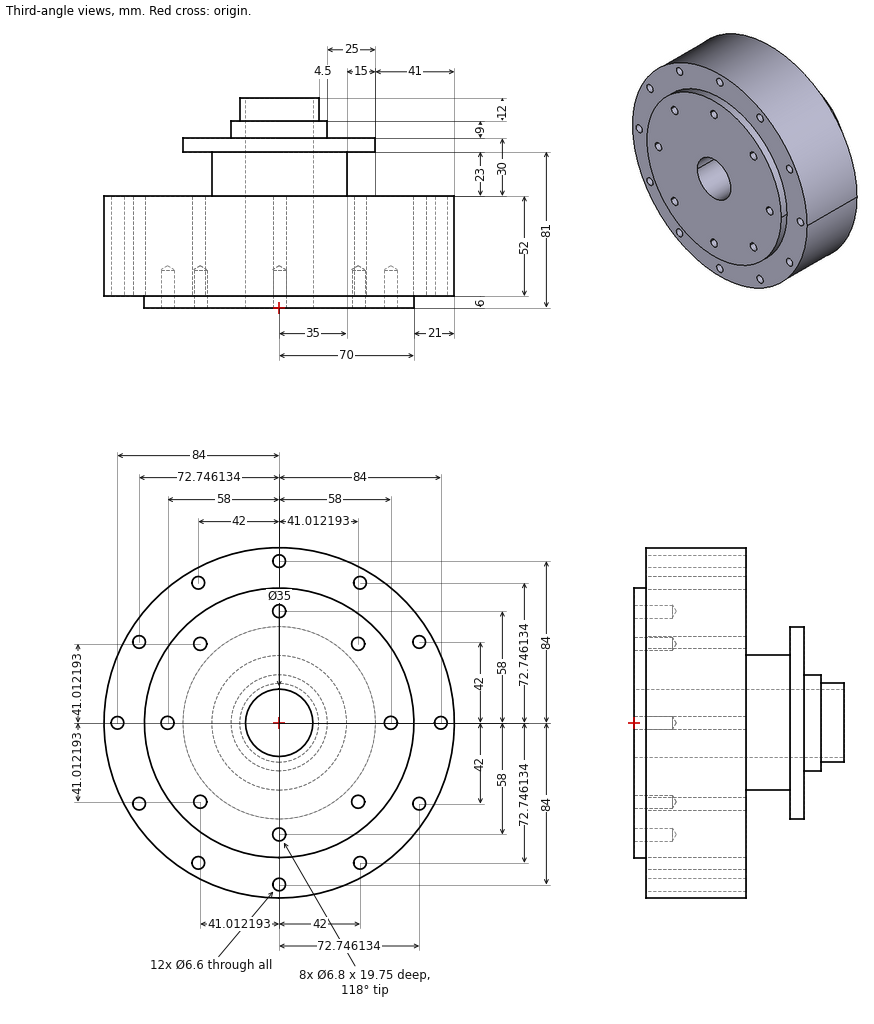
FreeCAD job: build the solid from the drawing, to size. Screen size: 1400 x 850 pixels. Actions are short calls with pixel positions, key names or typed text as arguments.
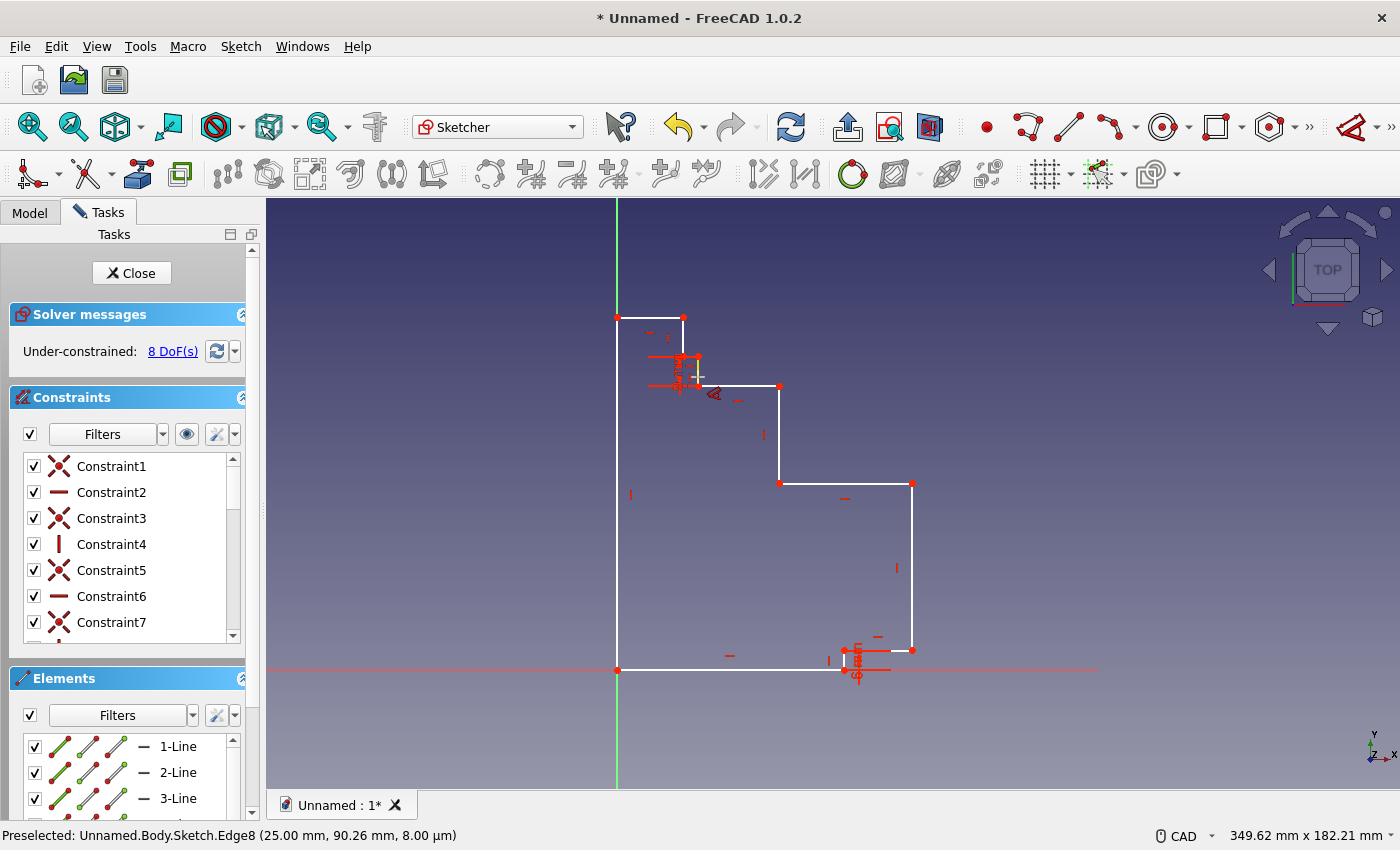
click(685, 670)
click(731, 704)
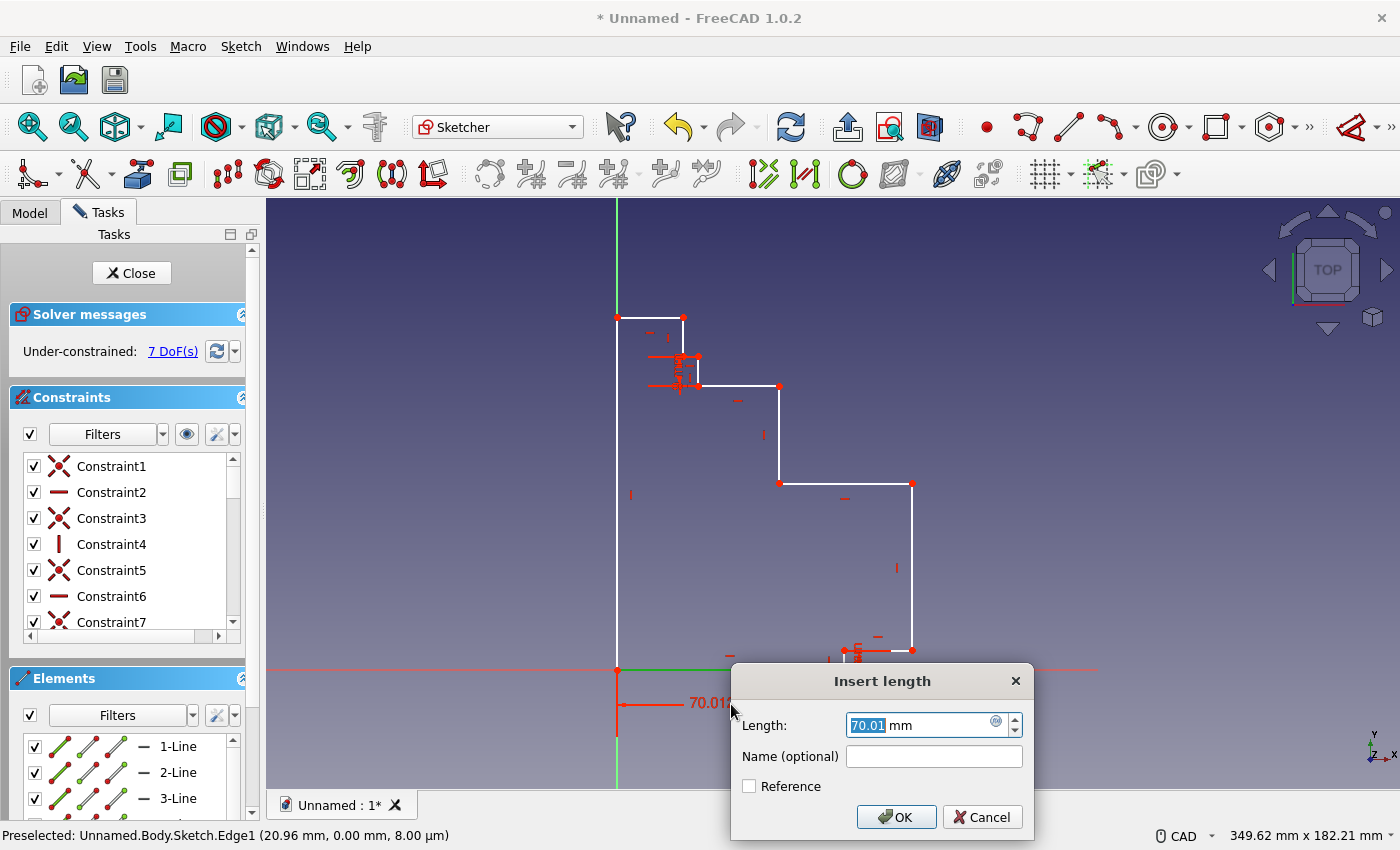
text(70)
key(Return)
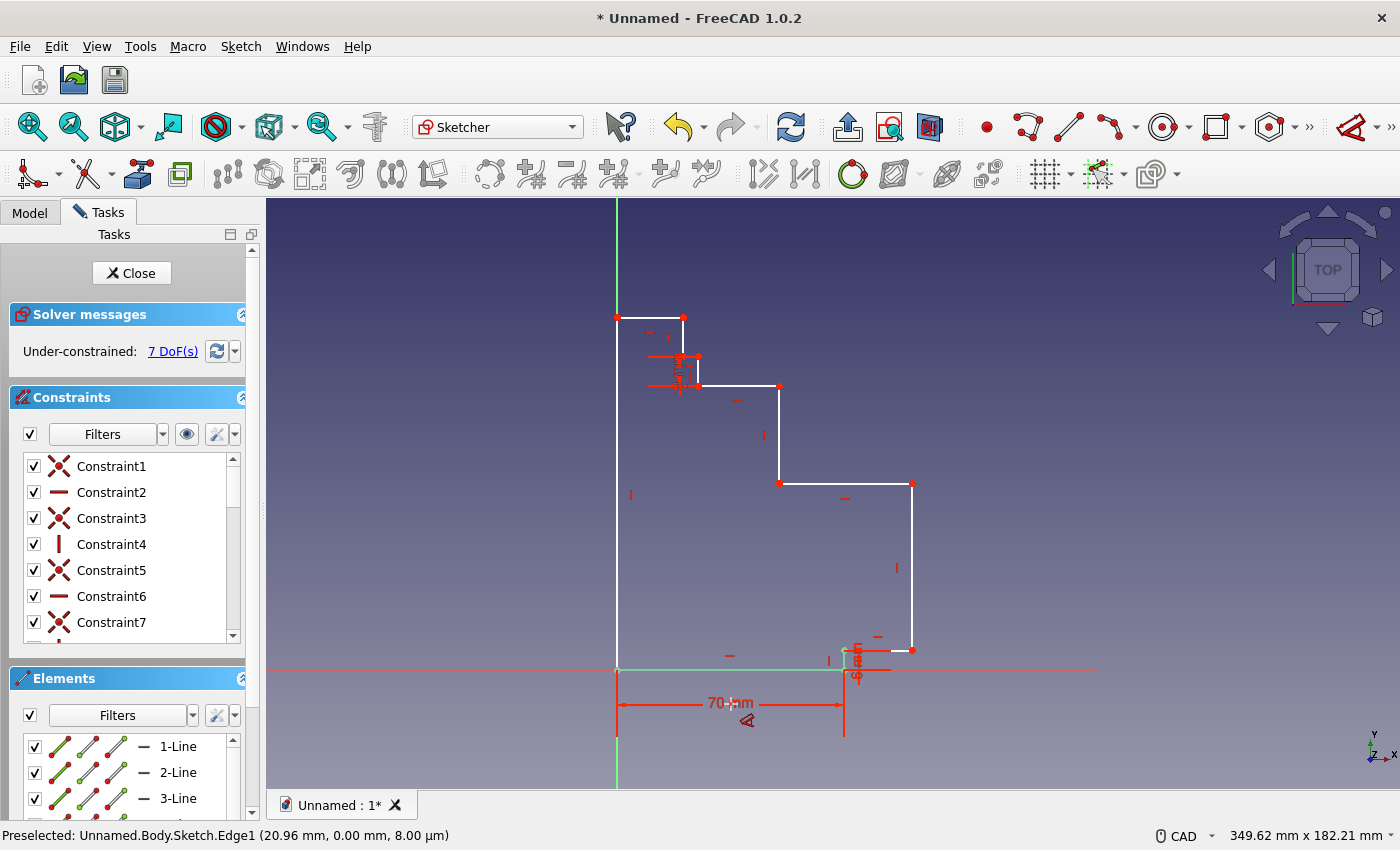
click(864, 651)
click(878, 685)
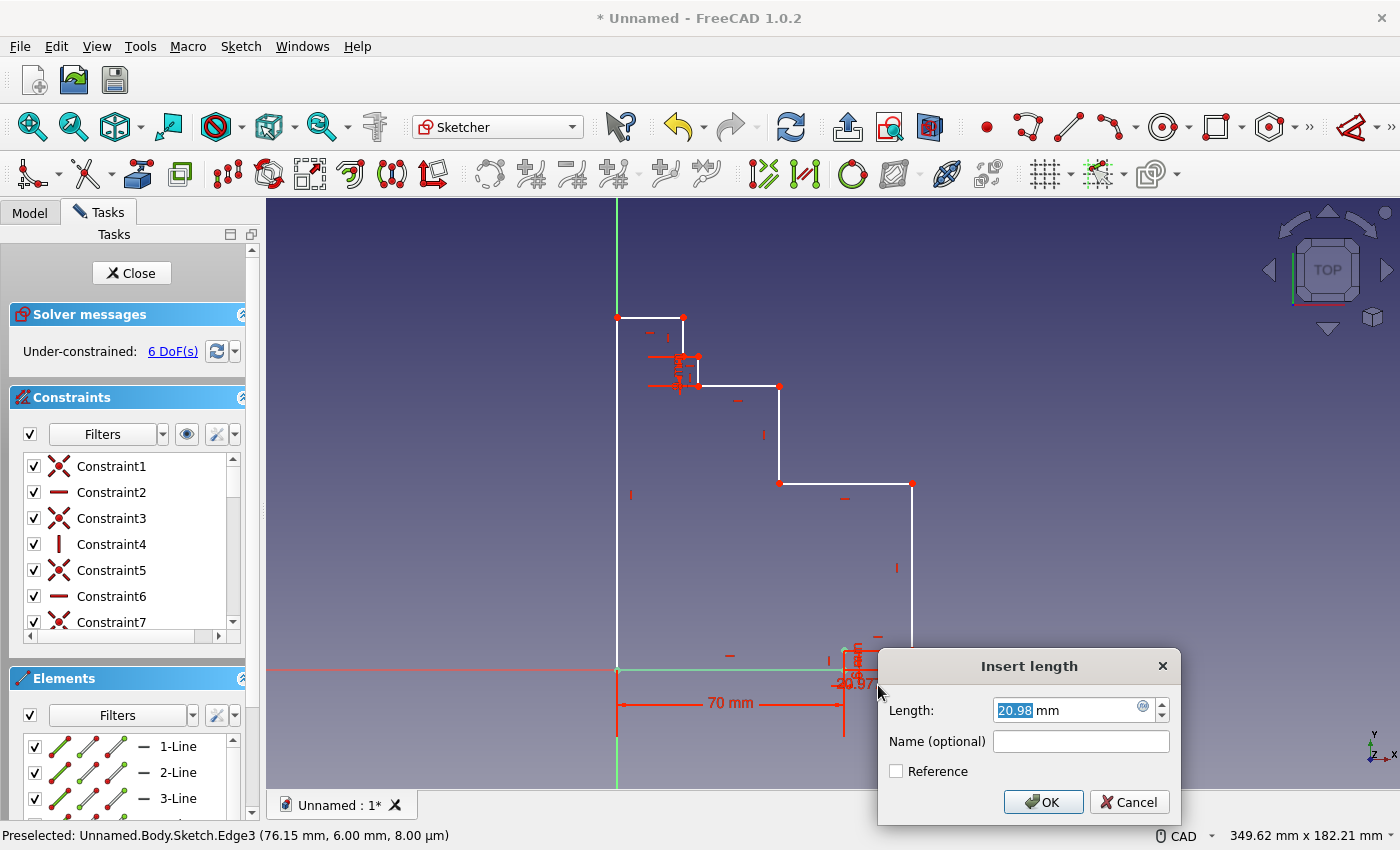
text(21)
key(Return)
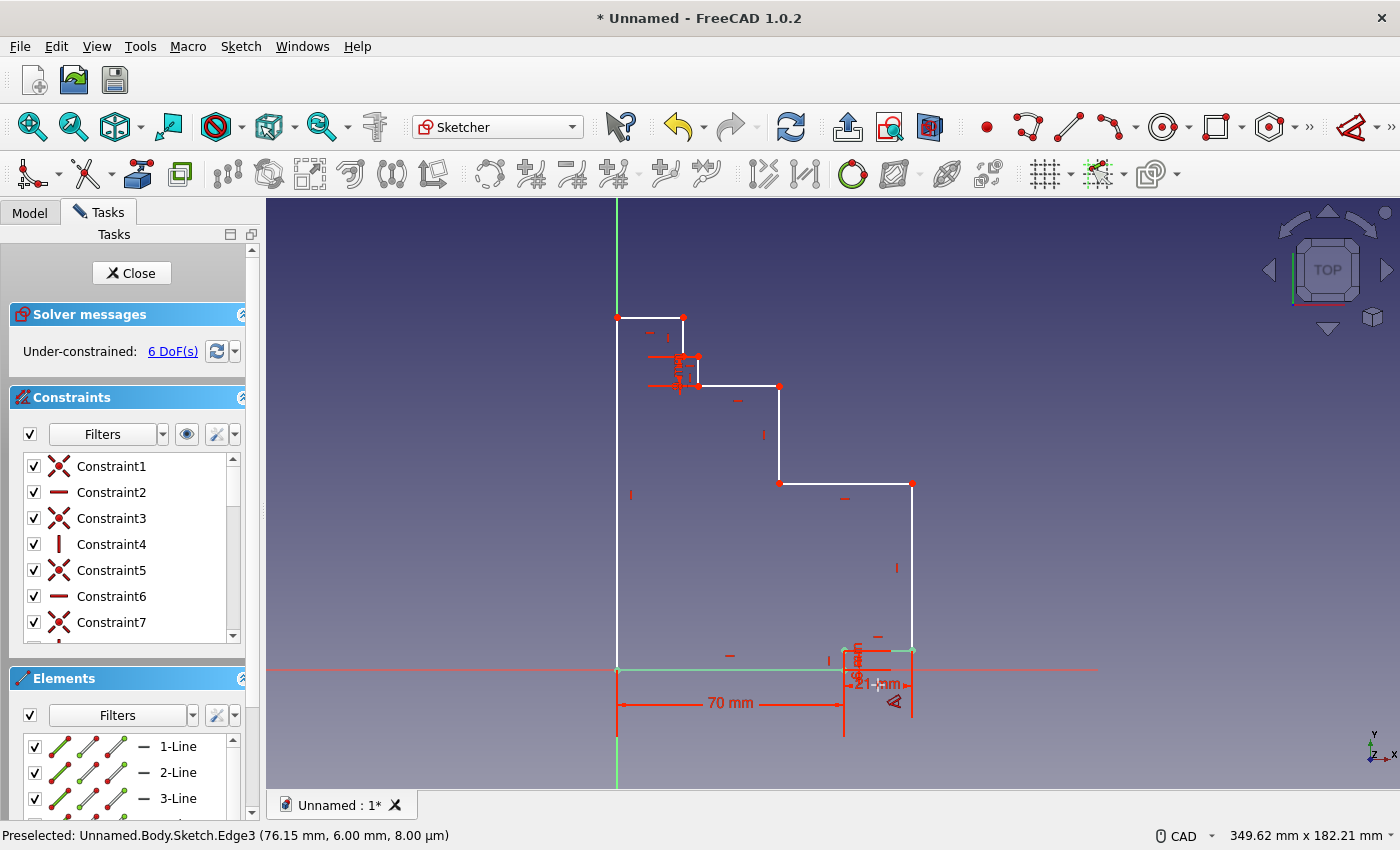
click(912, 601)
click(946, 567)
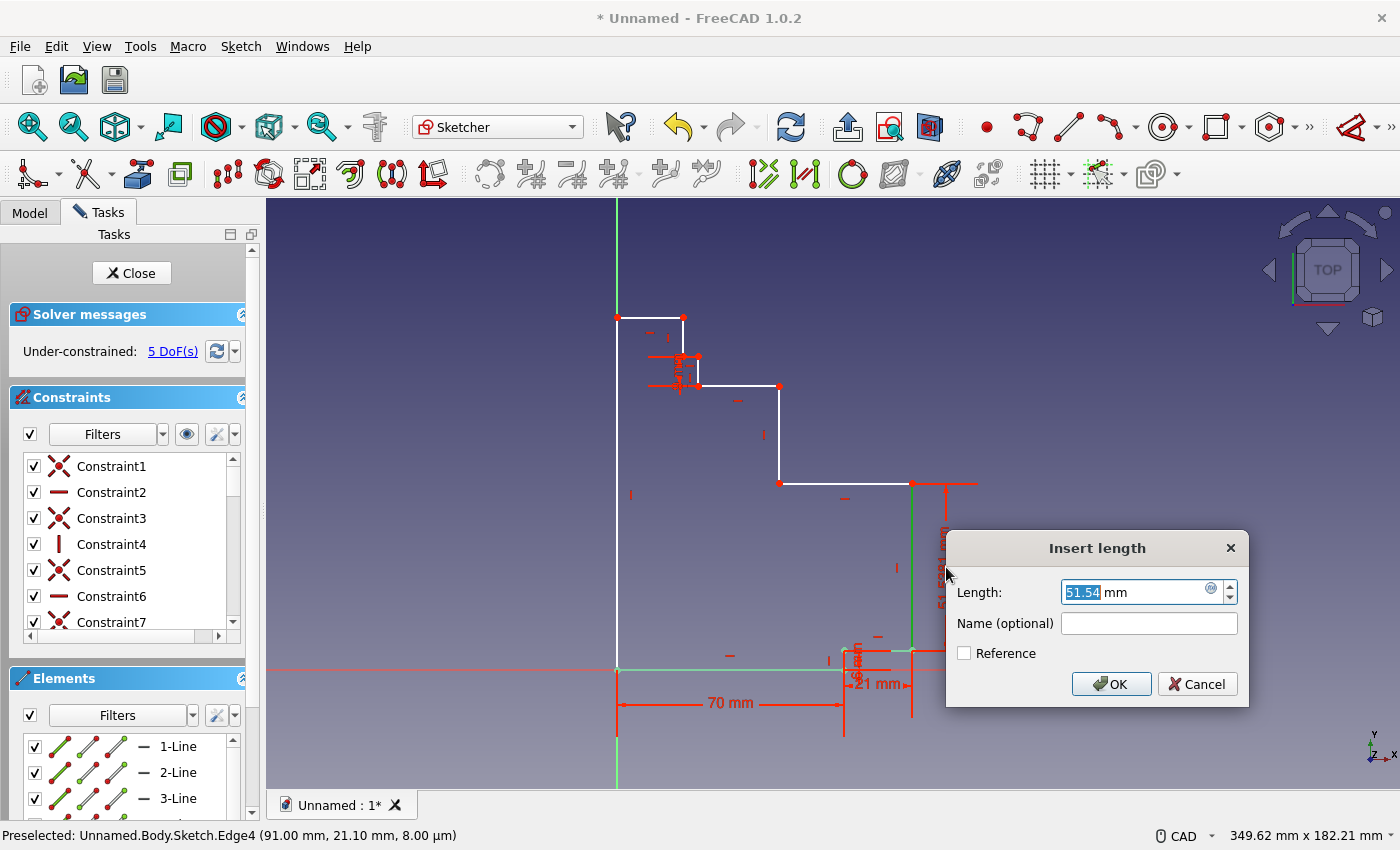
text(52)
key(Return)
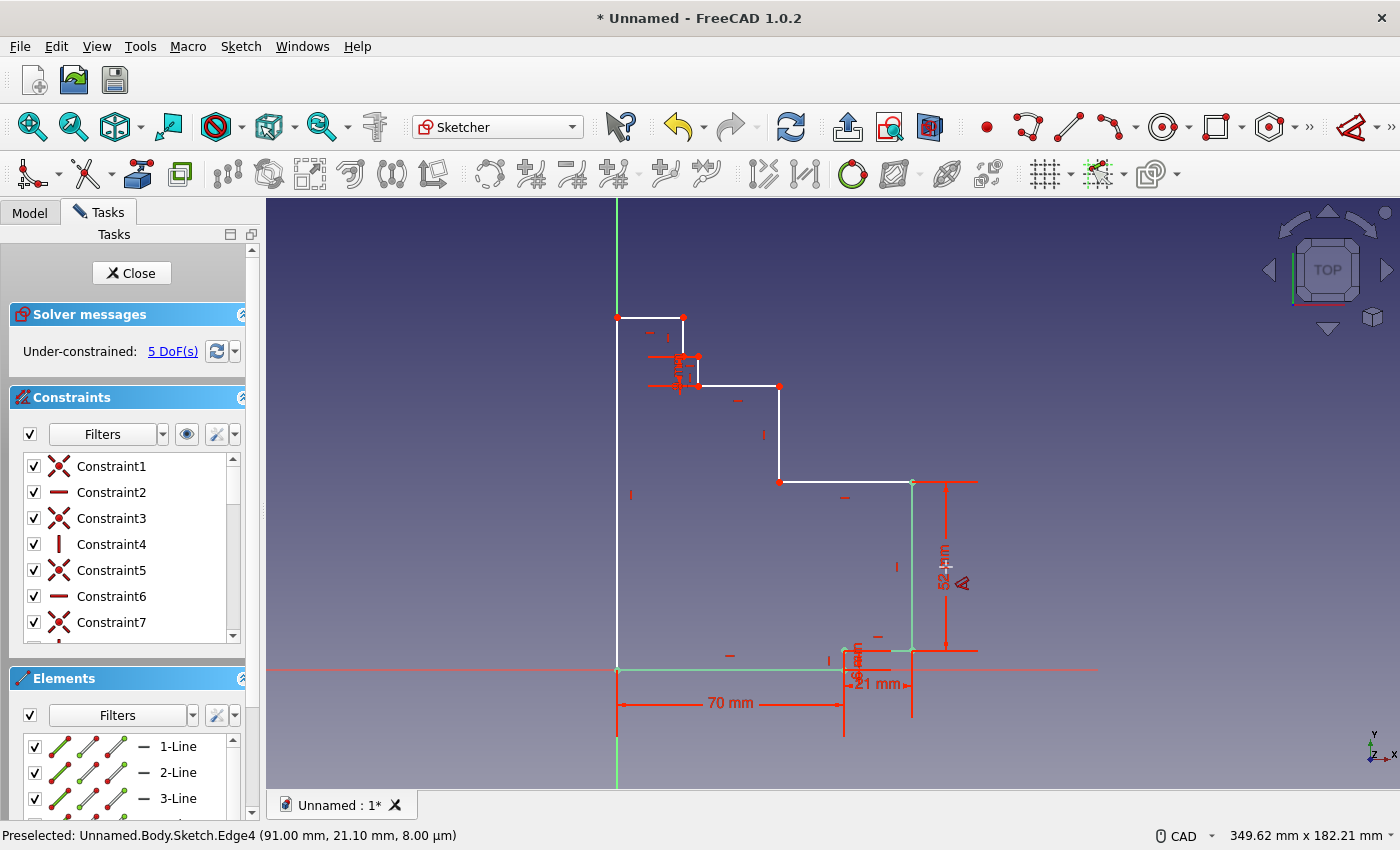
click(872, 482)
click(846, 448)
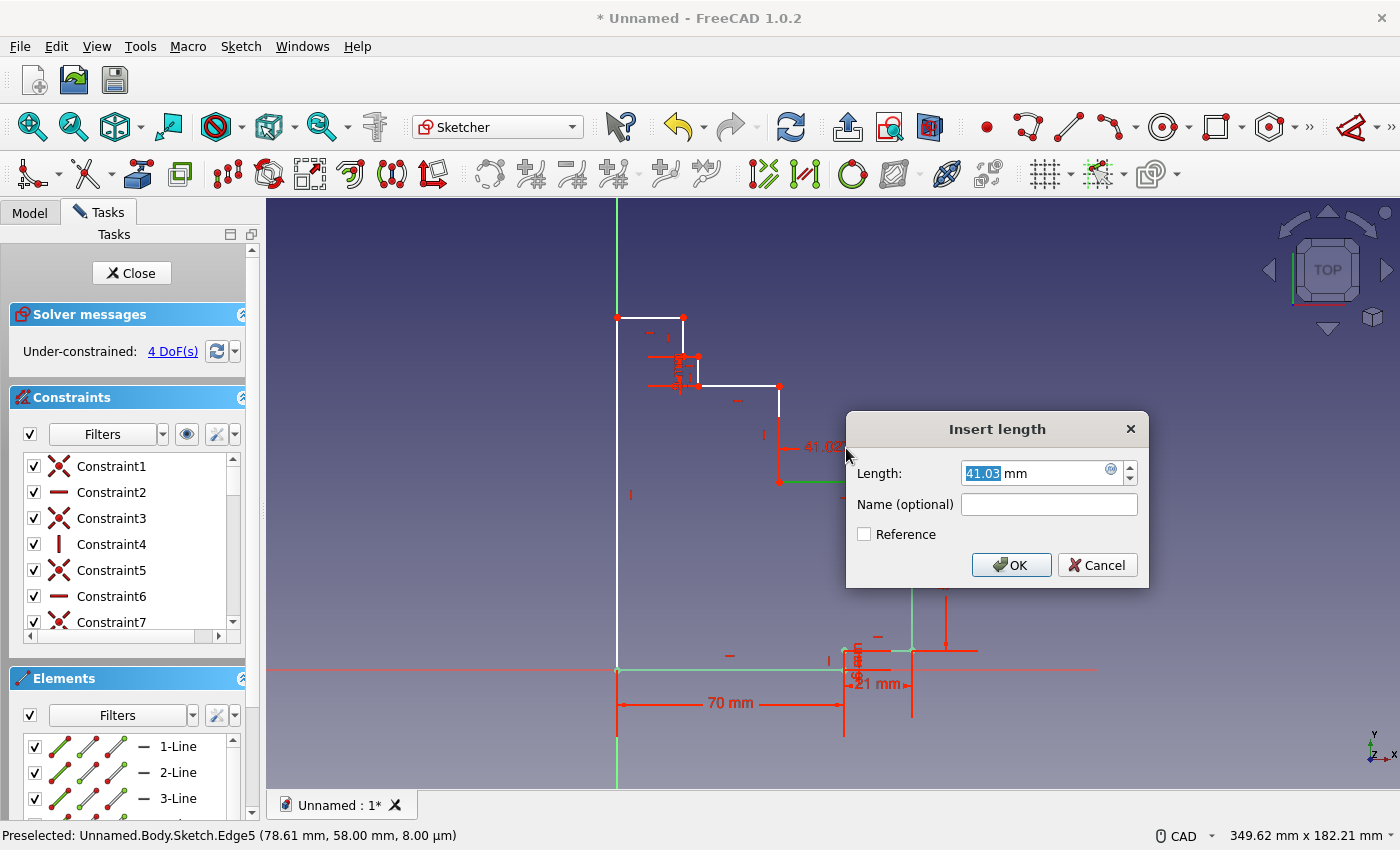
text(41)
key(Return)